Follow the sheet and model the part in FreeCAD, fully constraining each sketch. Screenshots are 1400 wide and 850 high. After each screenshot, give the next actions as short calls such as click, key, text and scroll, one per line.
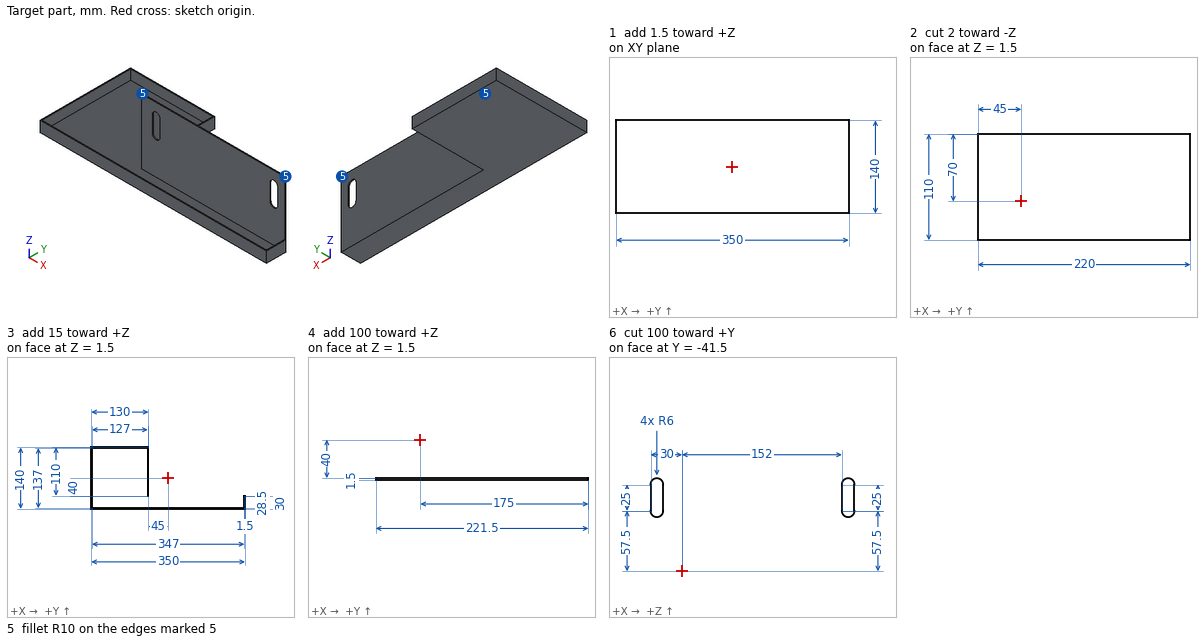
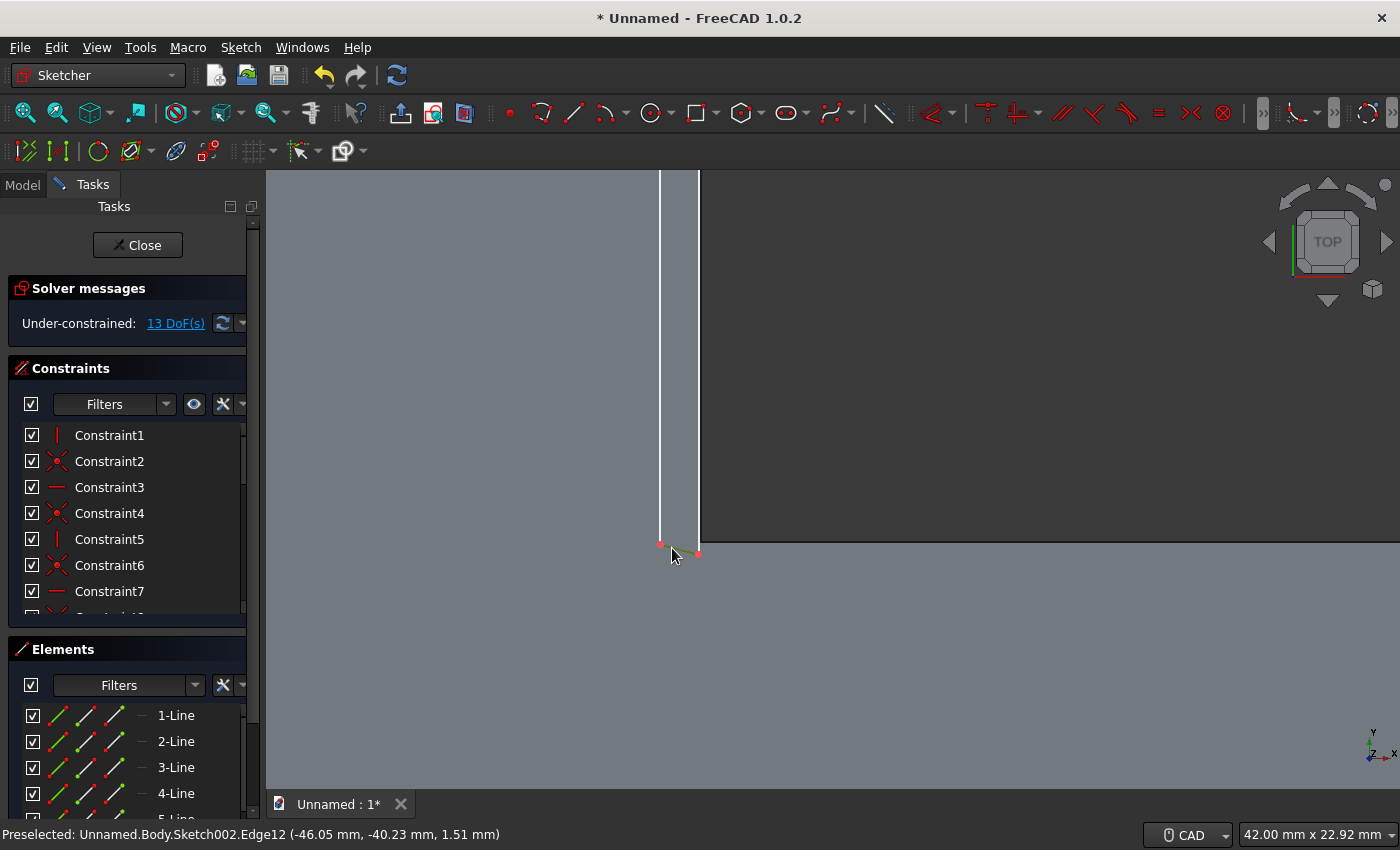
click(1040, 114)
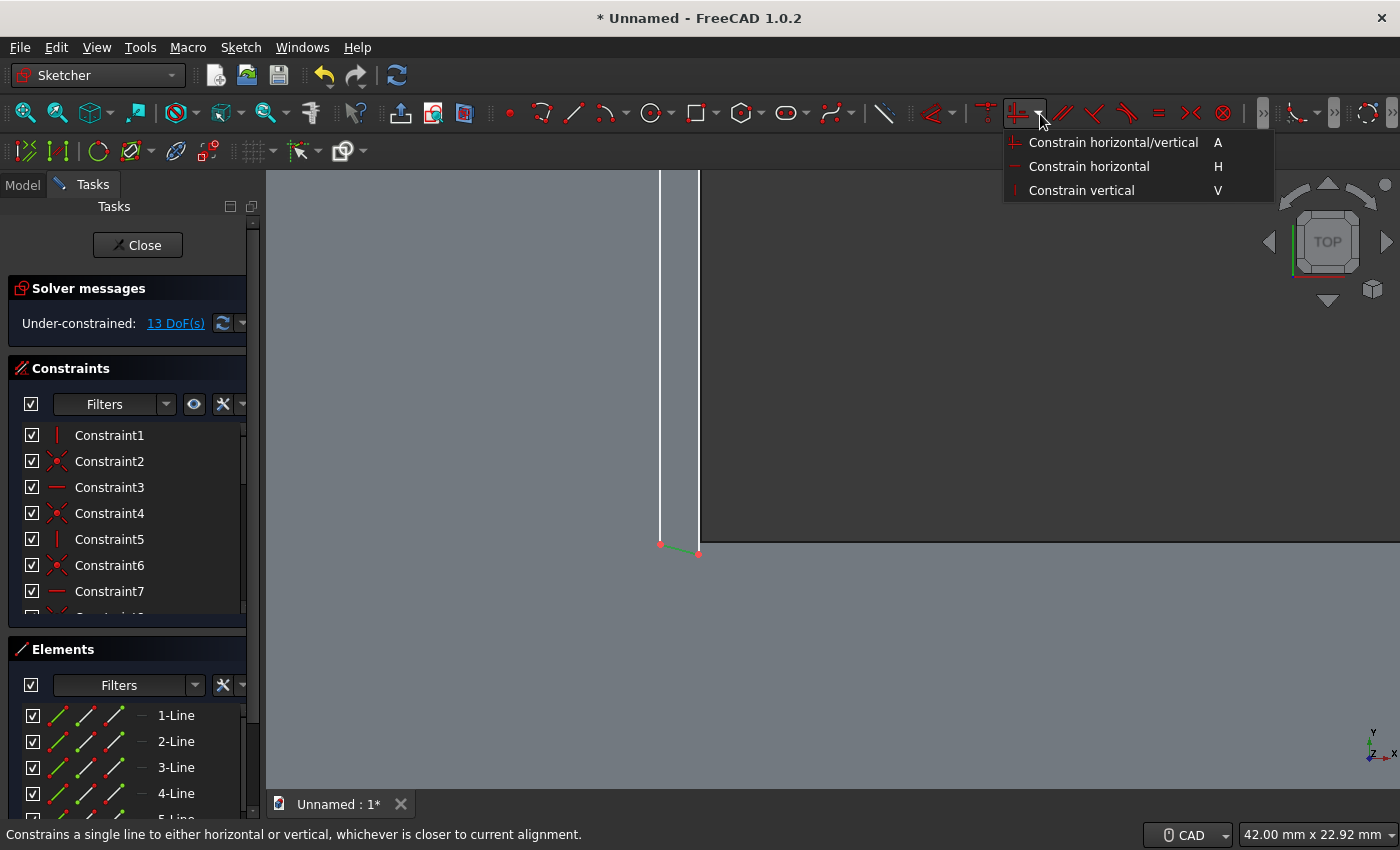
click(1139, 166)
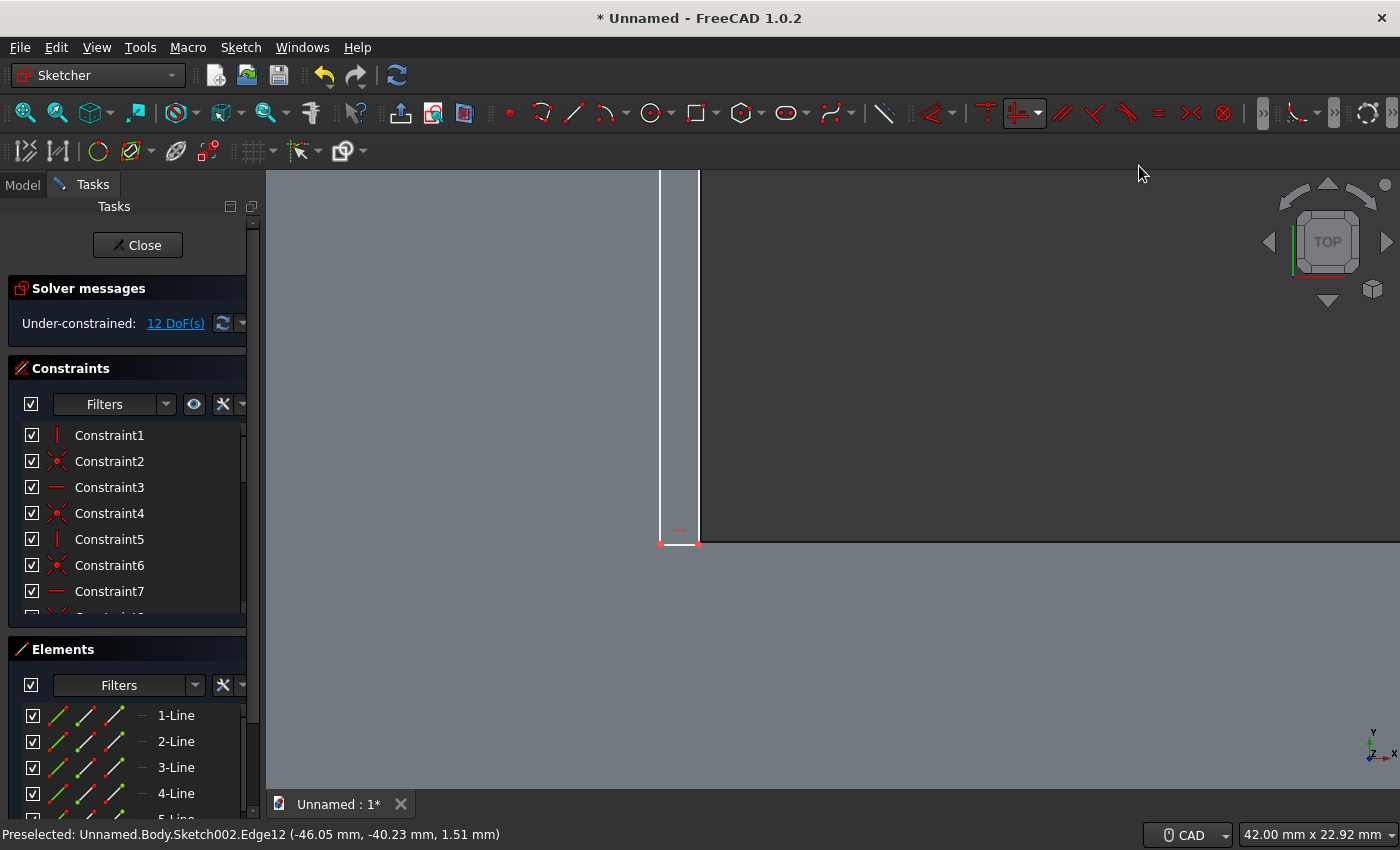
click(932, 114)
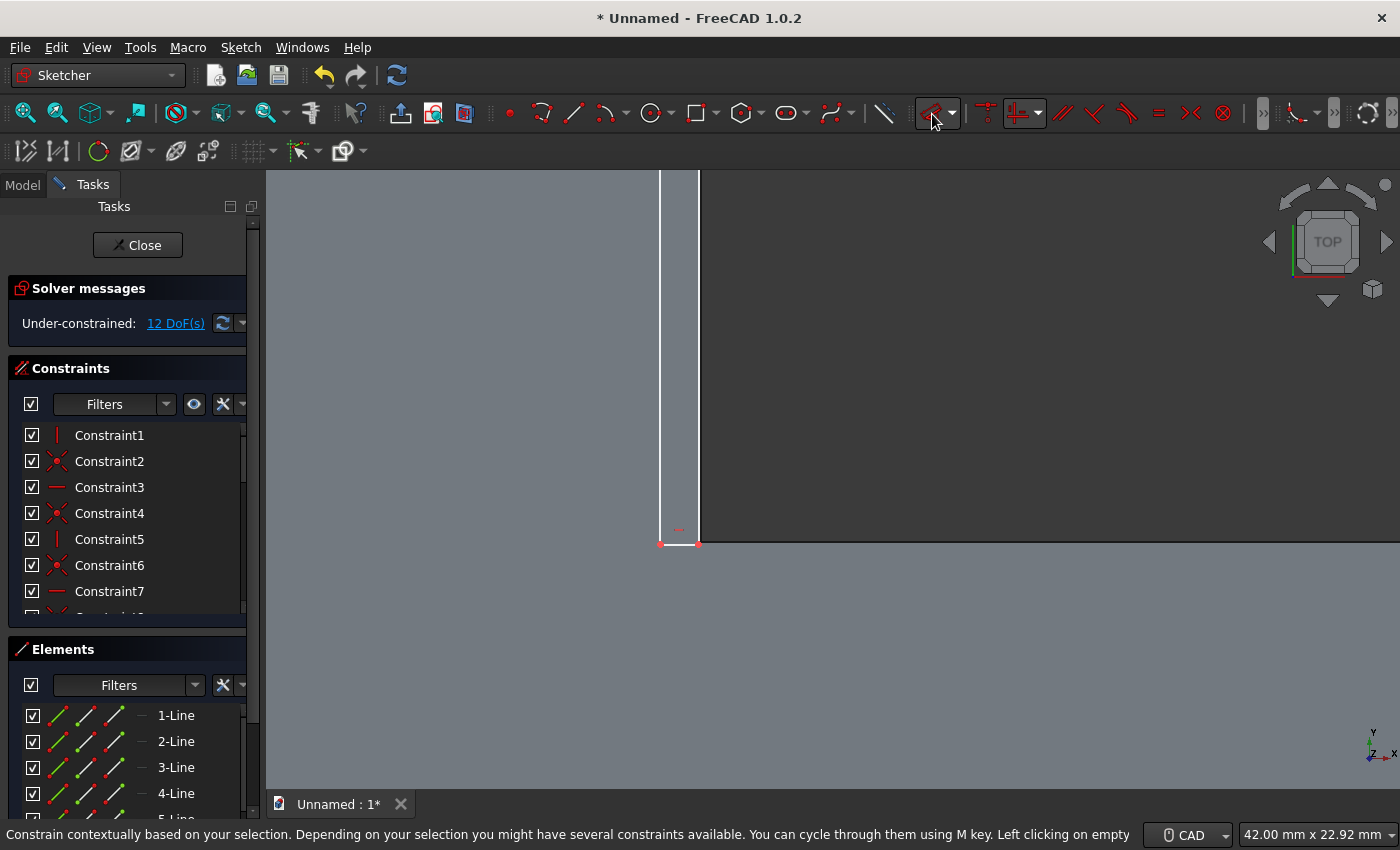
scroll(672, 561, down, 13)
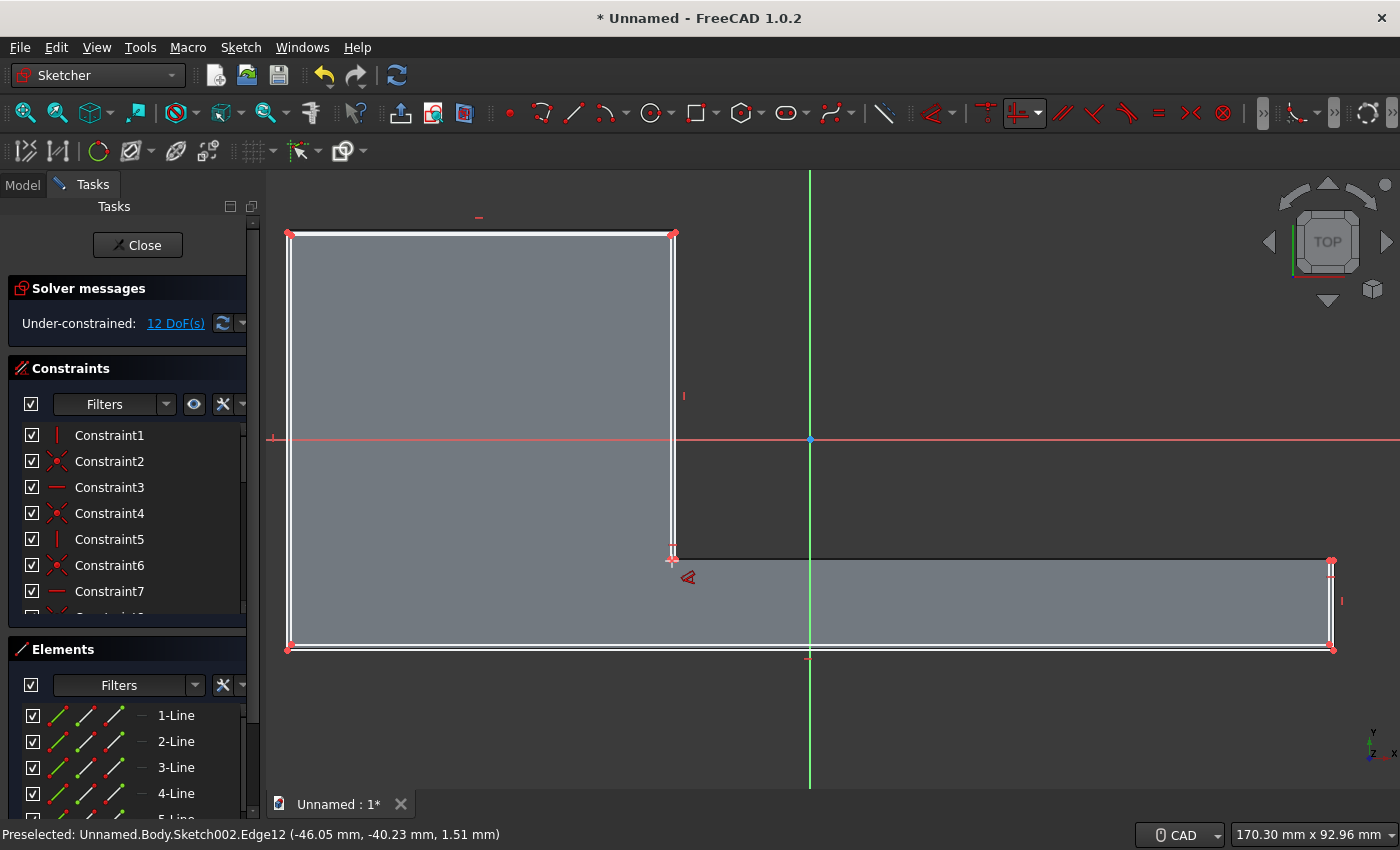
scroll(1115, 603, up, 9)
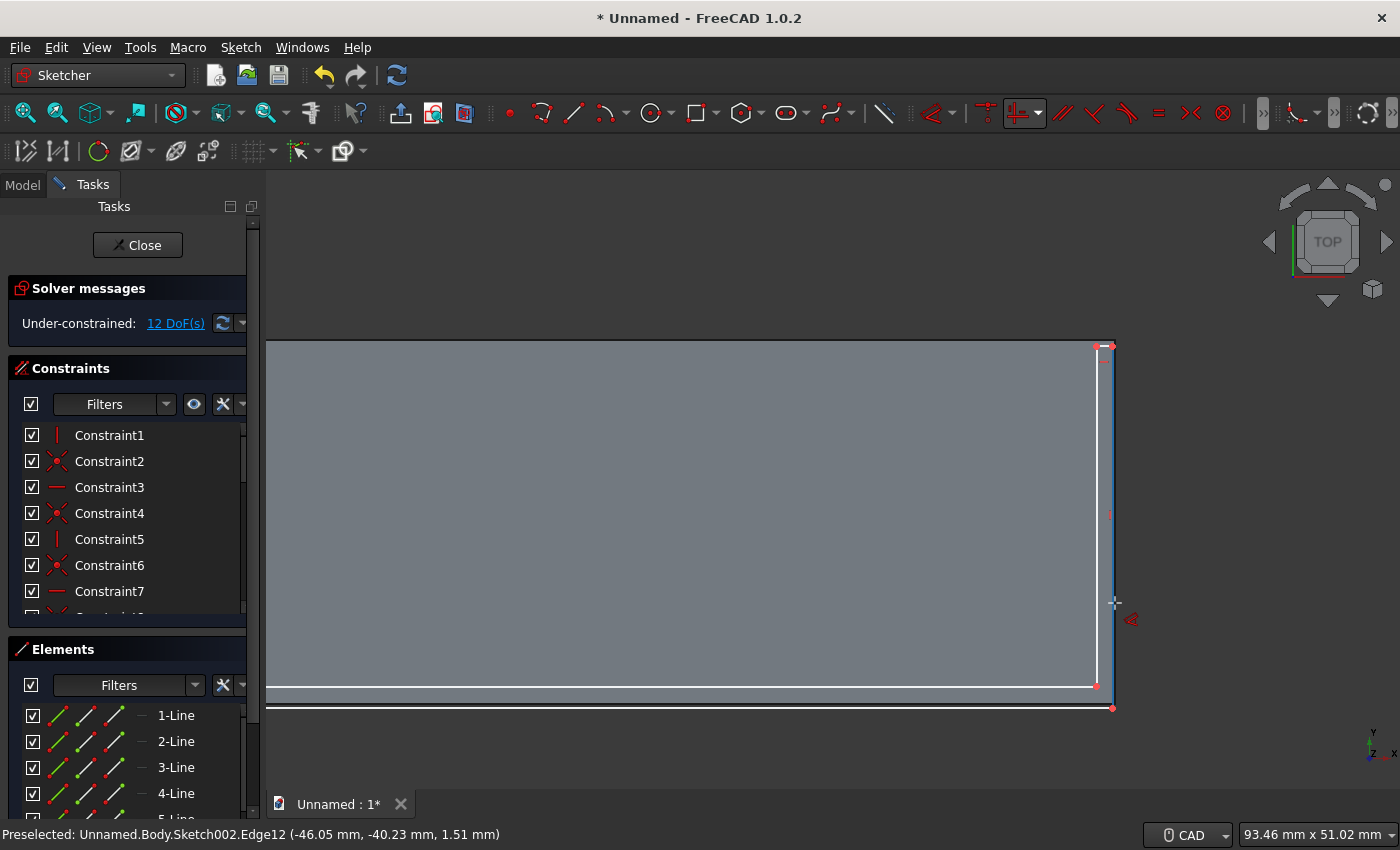
click(1113, 600)
click(1147, 527)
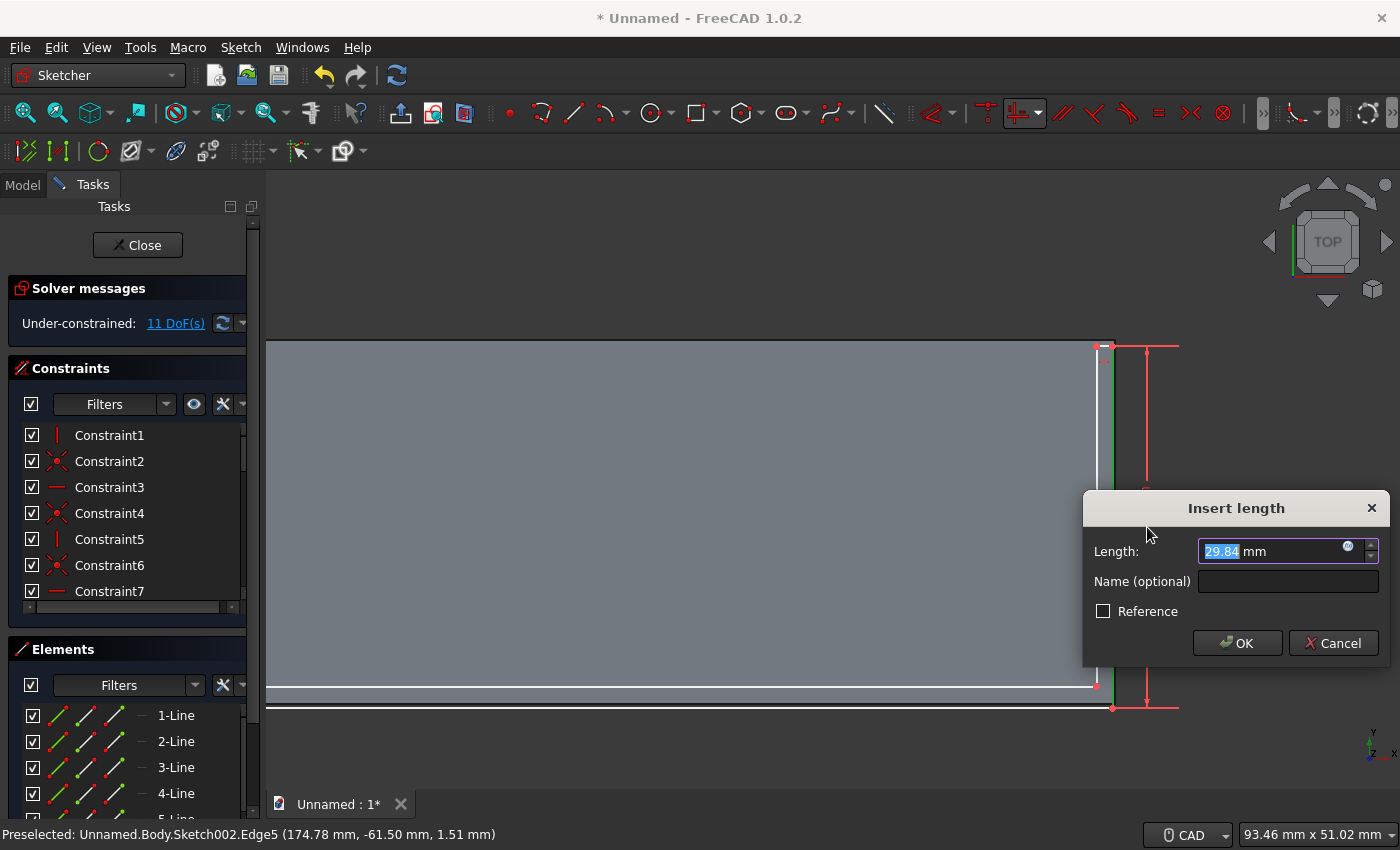
text(30)
key(Return)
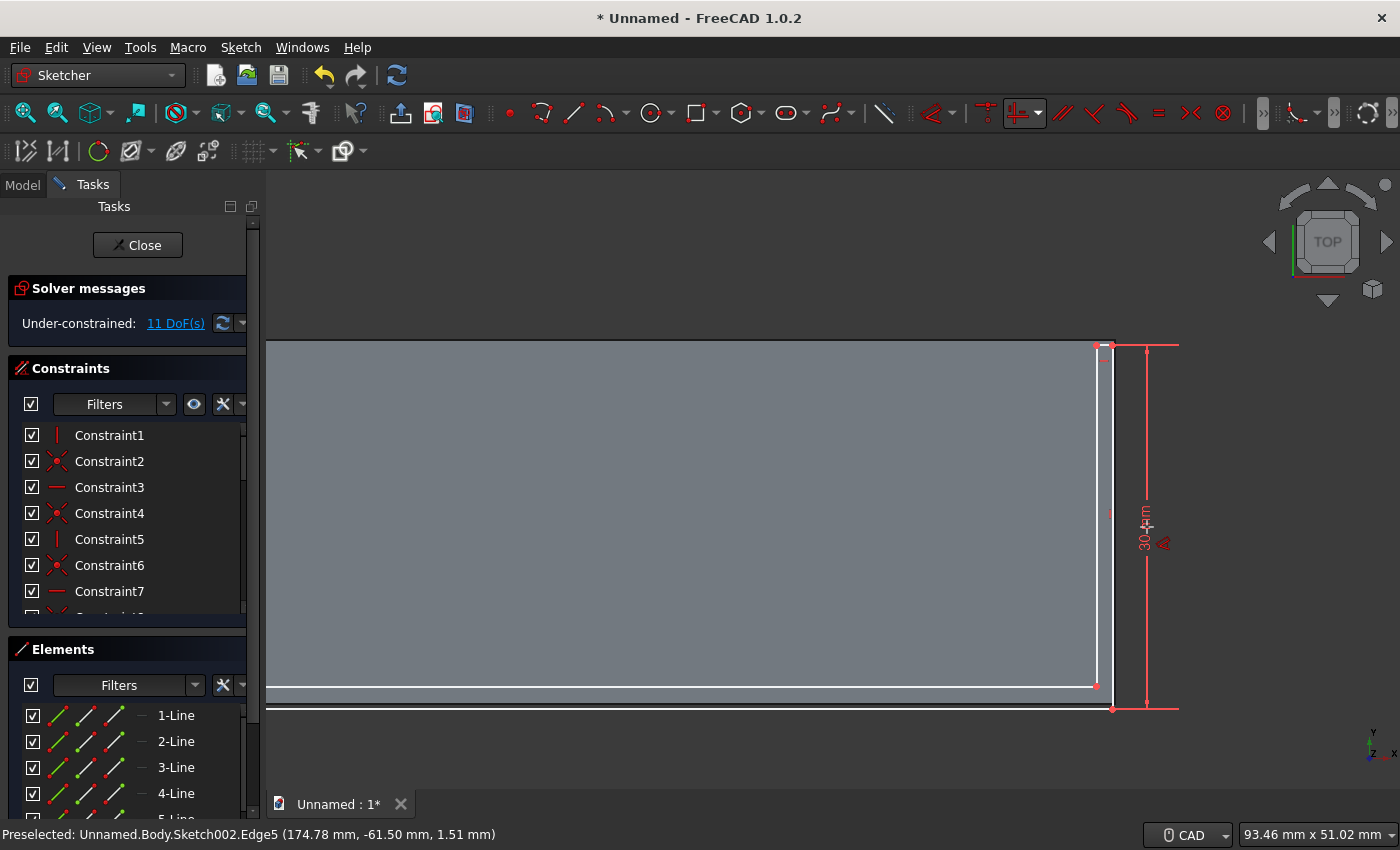
scroll(1116, 603, down, 9)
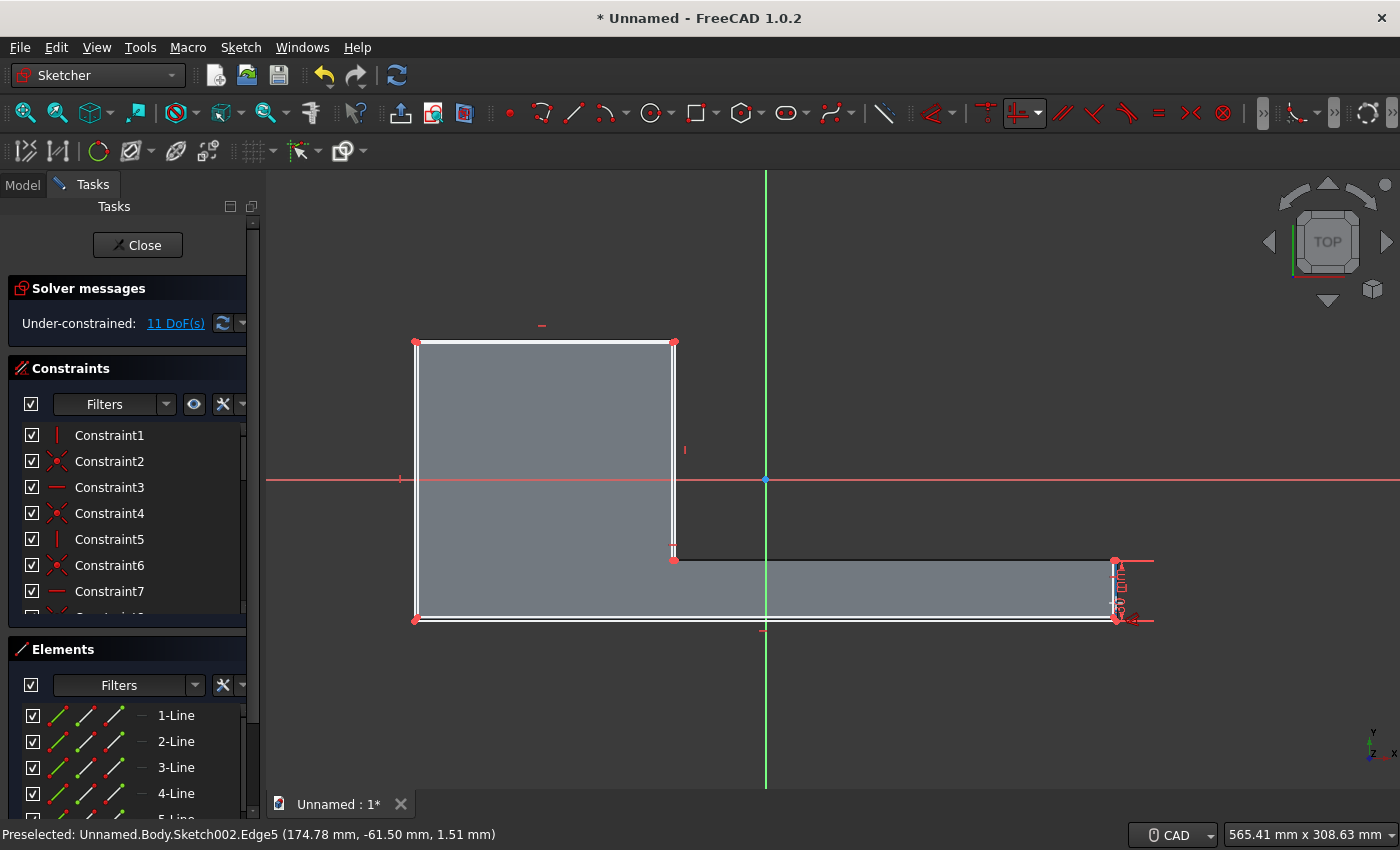
scroll(675, 495, up, 8)